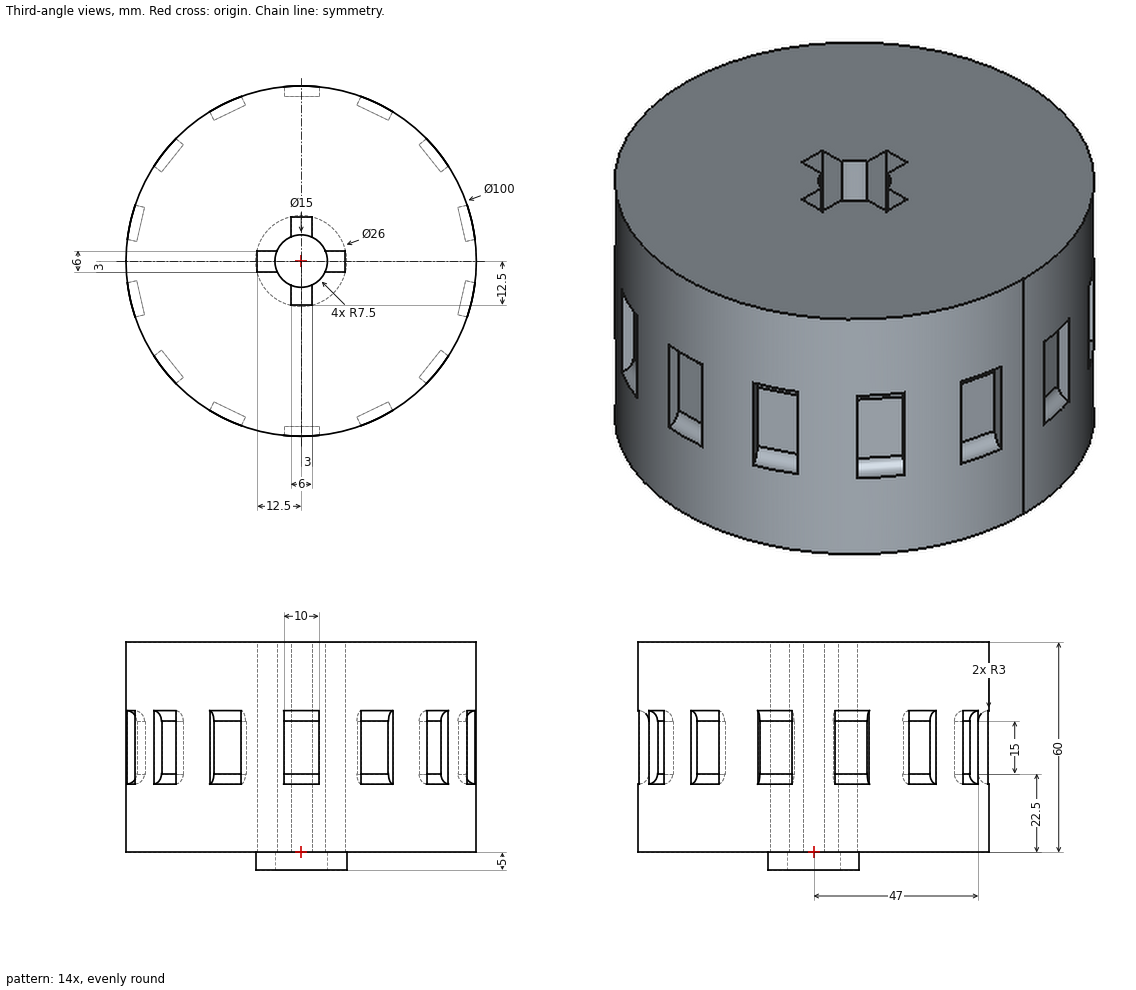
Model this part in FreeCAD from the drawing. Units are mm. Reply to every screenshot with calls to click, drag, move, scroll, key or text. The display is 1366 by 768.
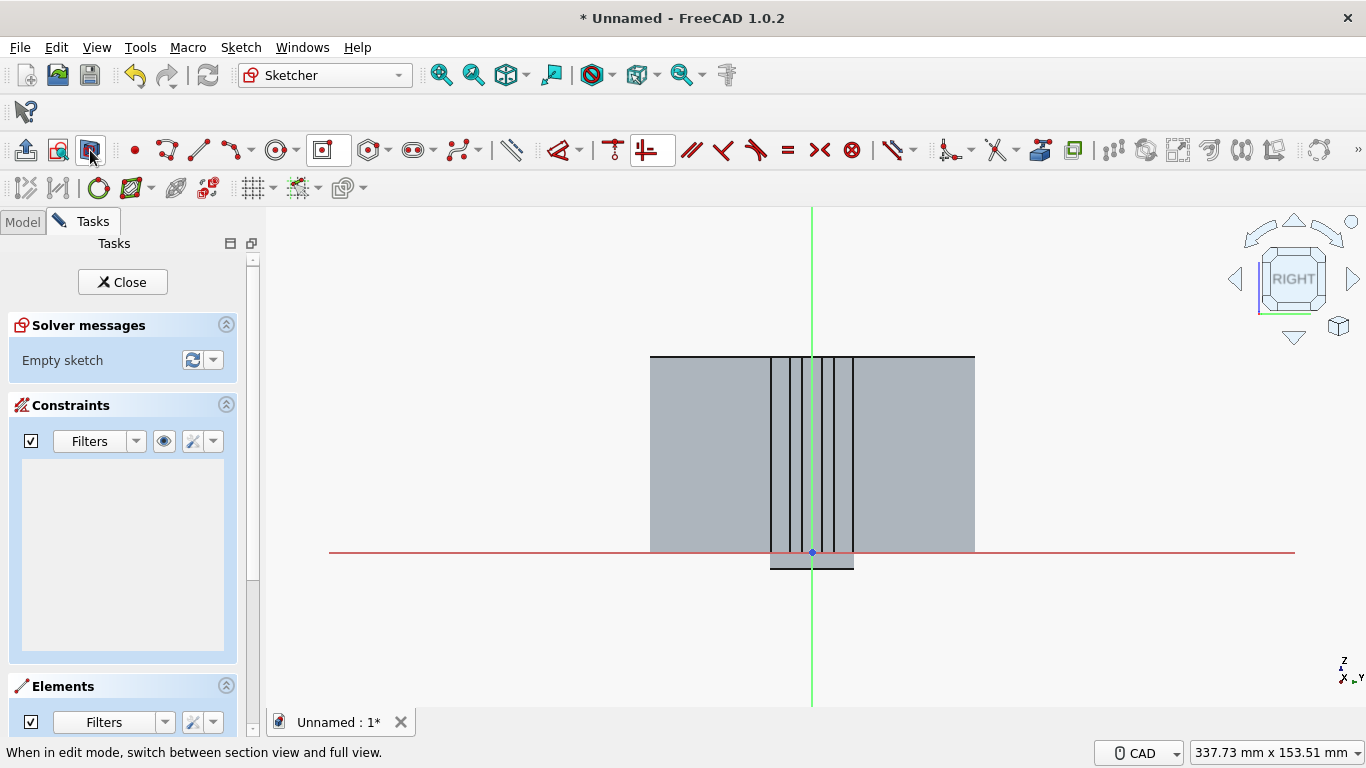
scroll(1032, 455, up, 8)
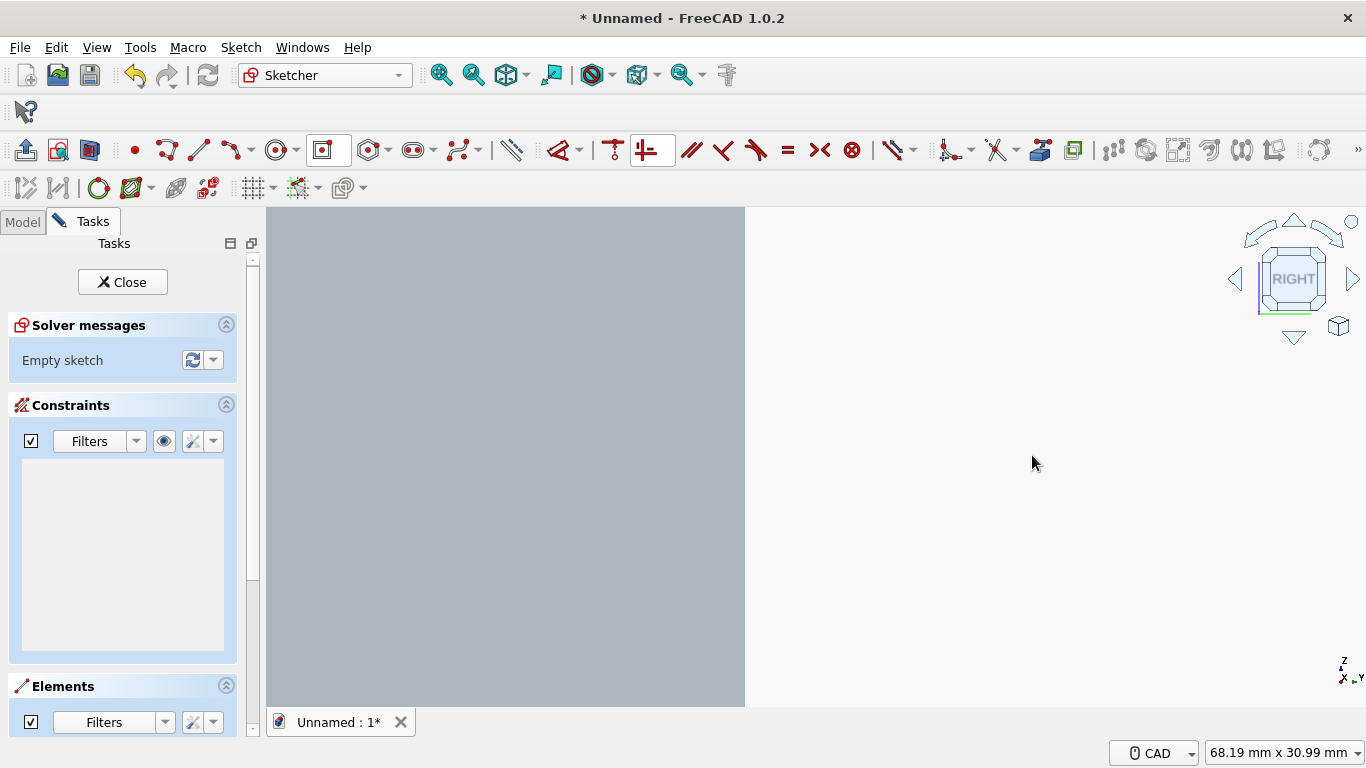
click(414, 150)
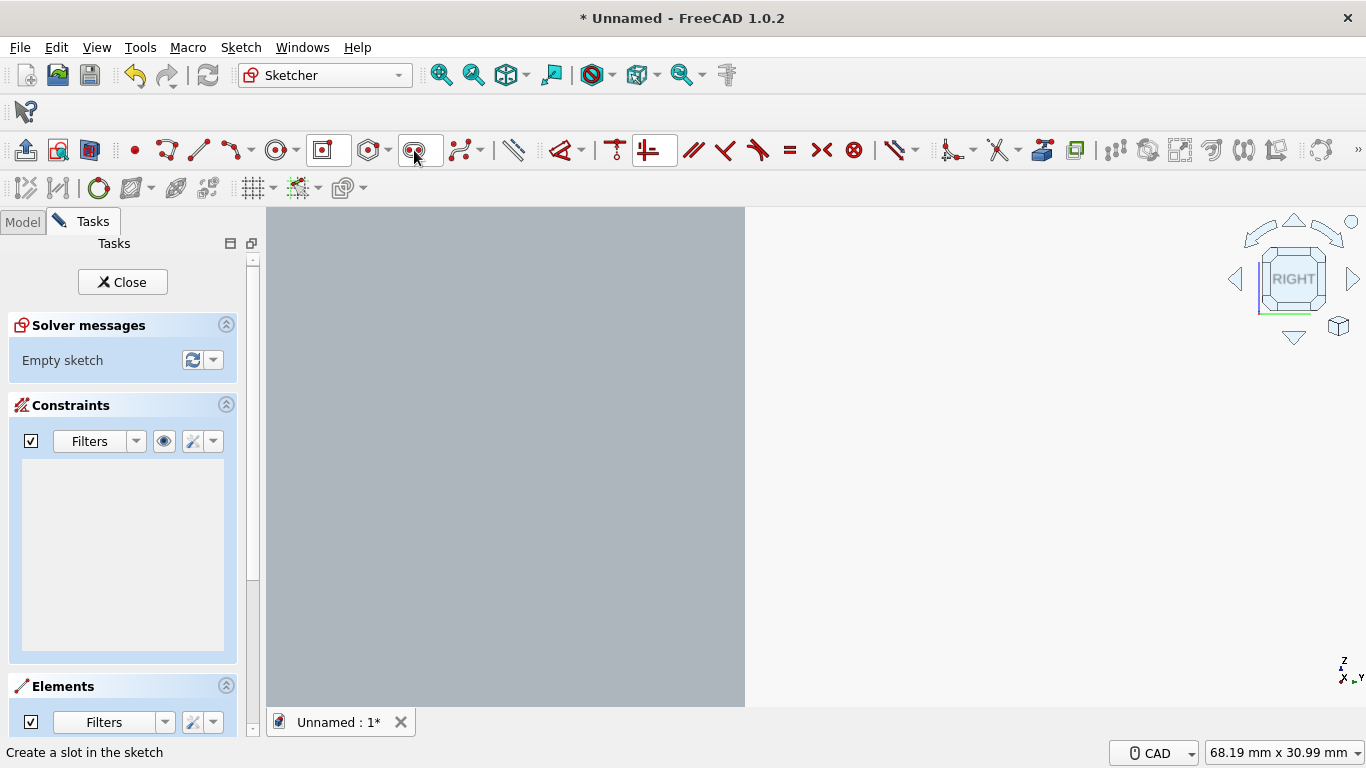
click(747, 575)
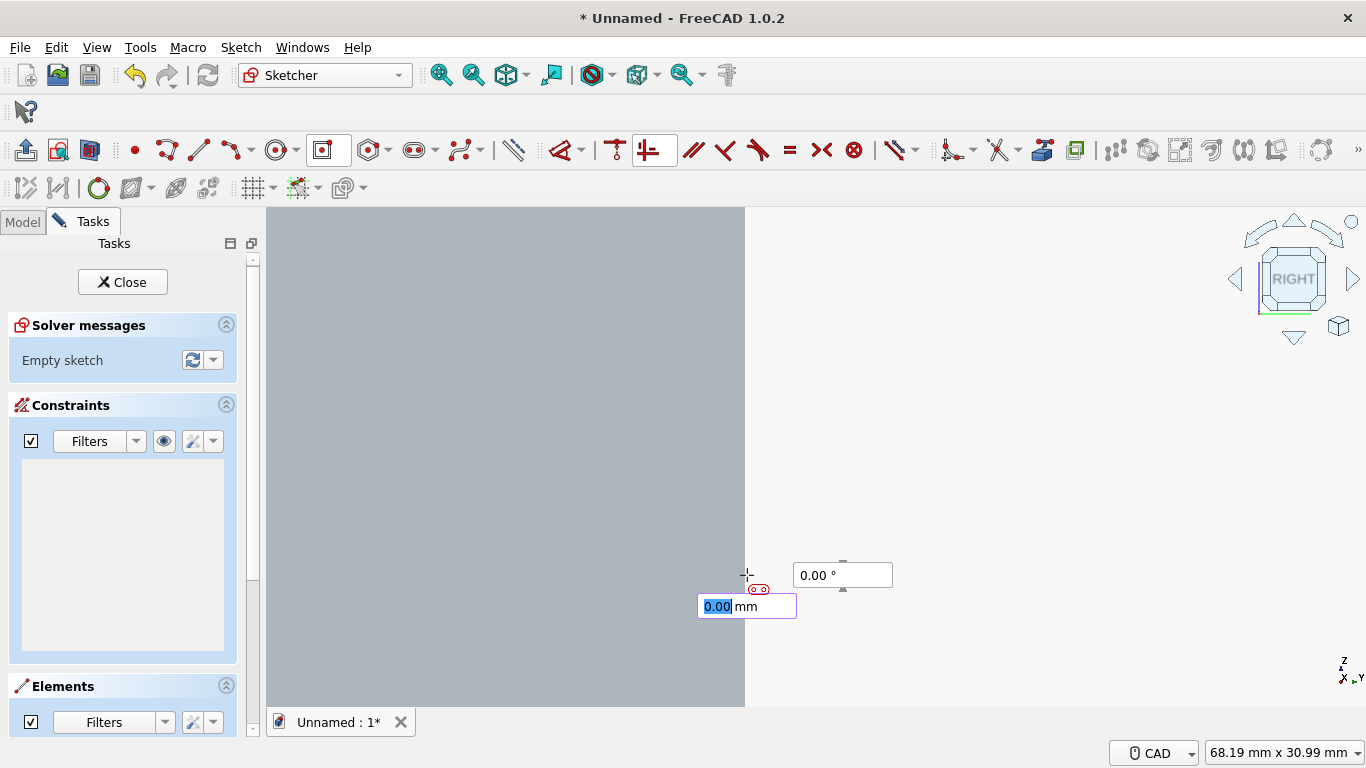
click(747, 333)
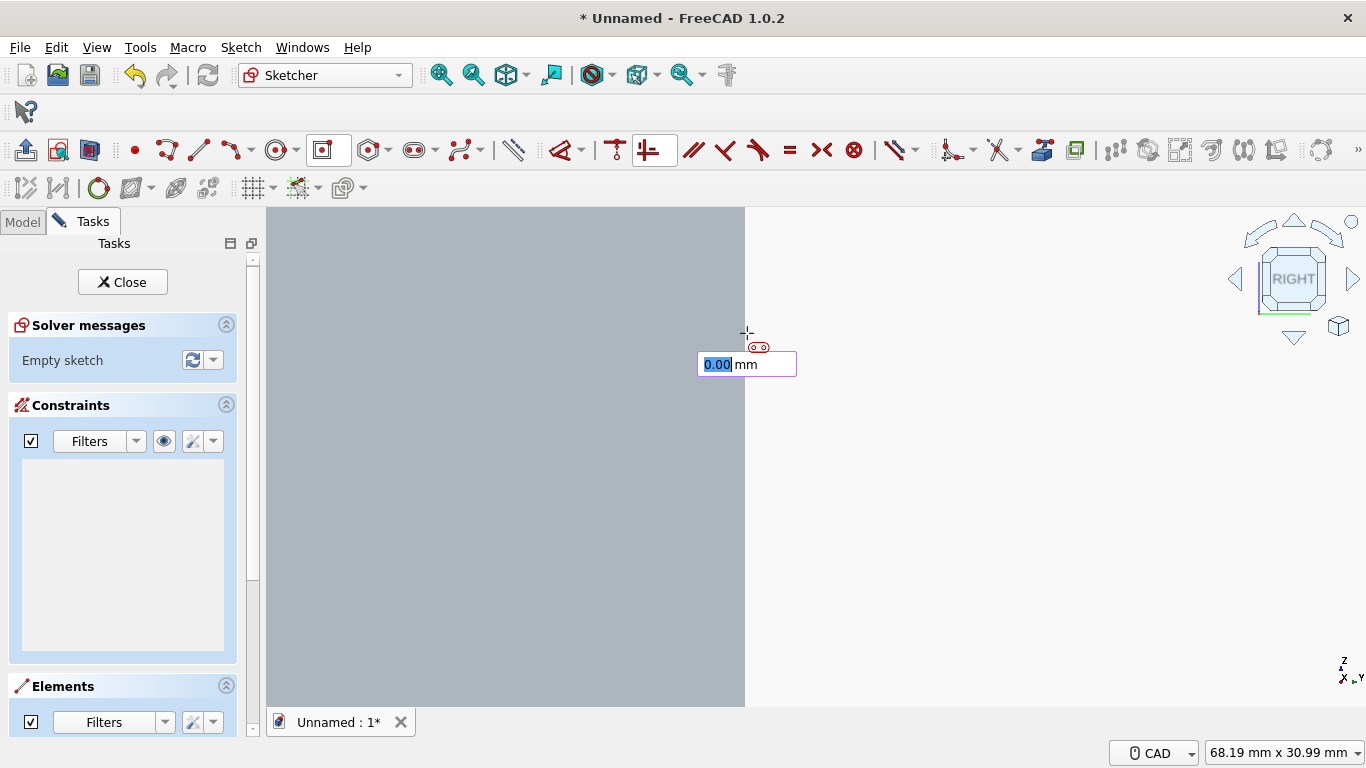
click(795, 454)
key(Escape)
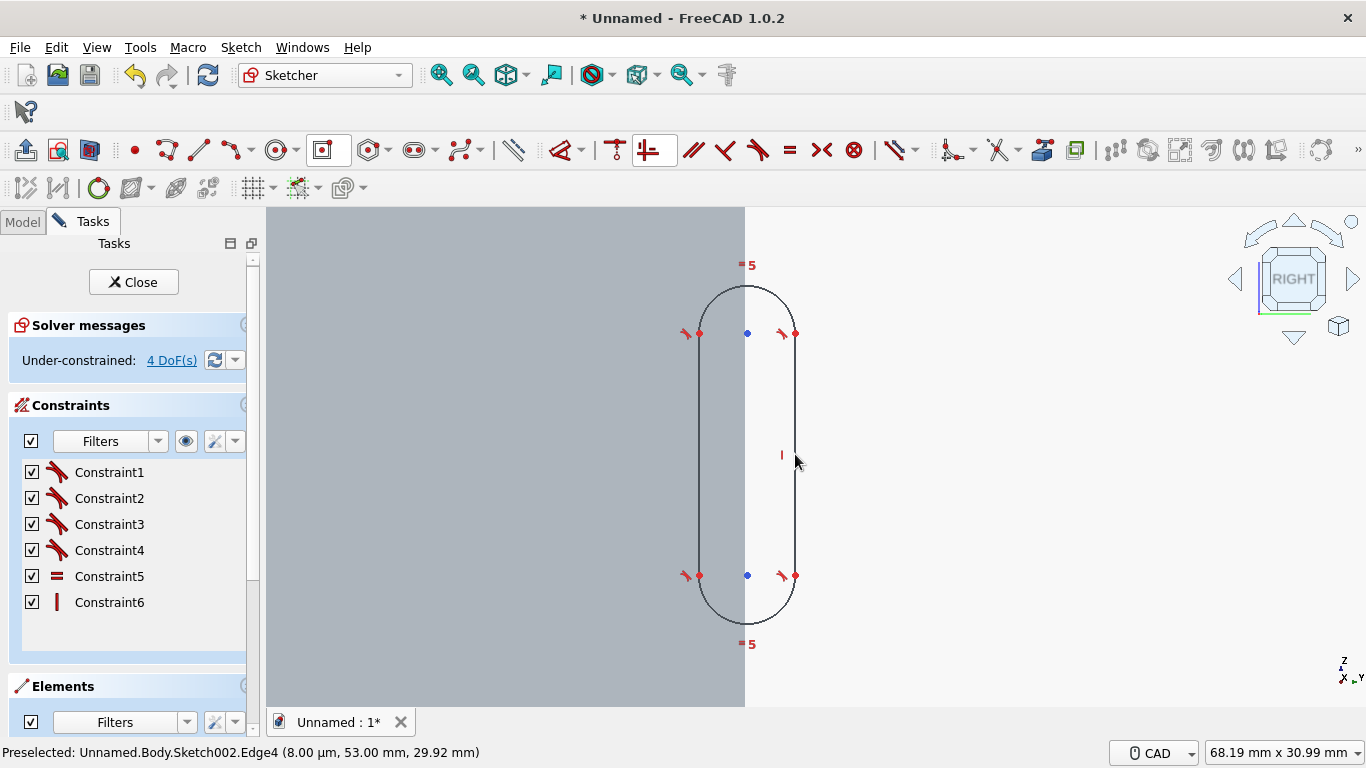
key(d)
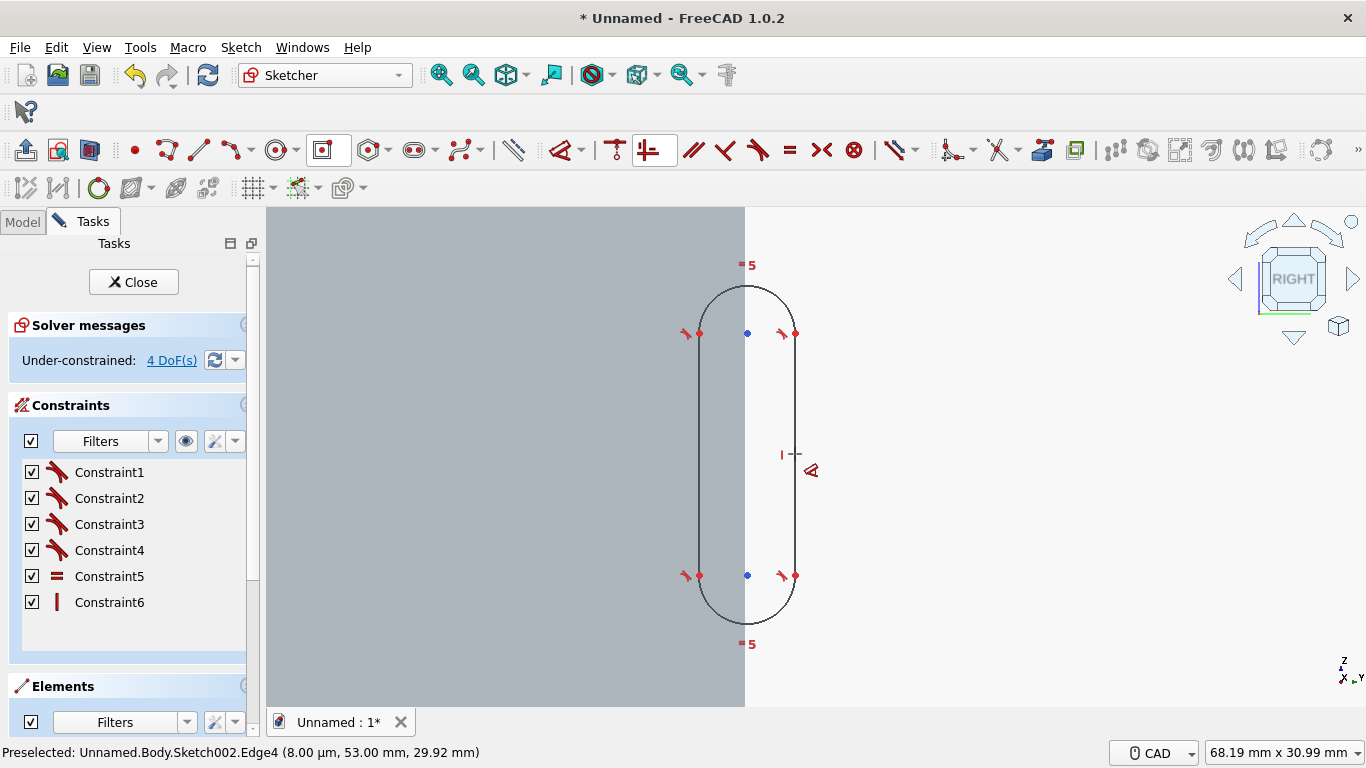
click(719, 615)
click(700, 641)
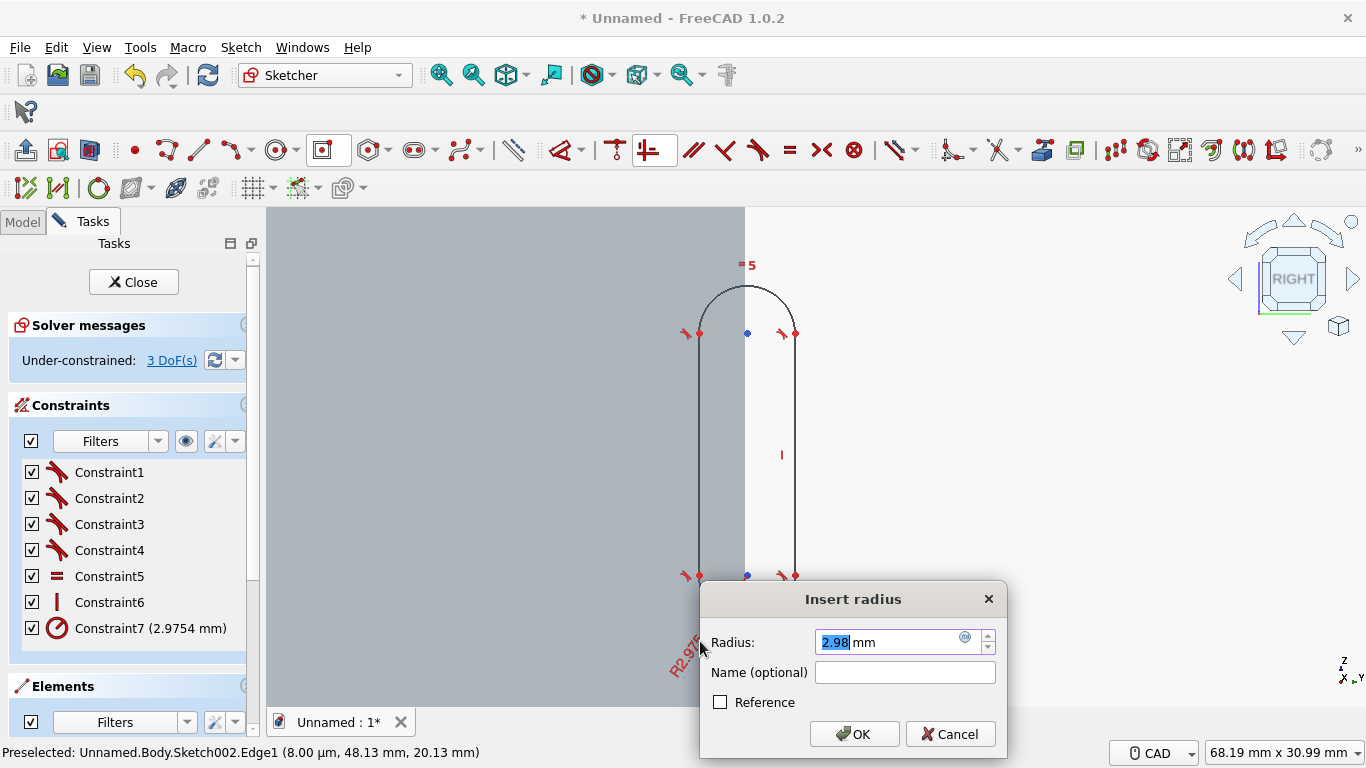
text(3)
key(Return)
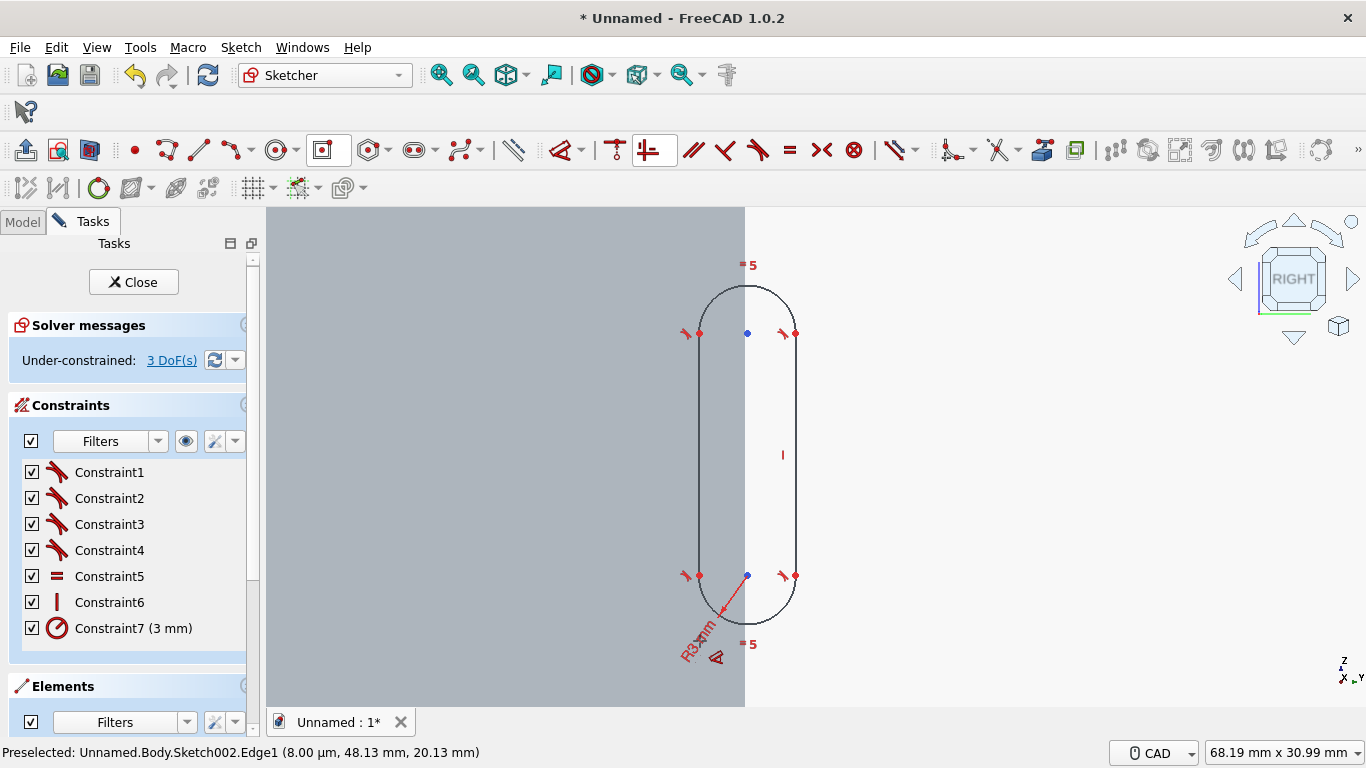
click(699, 503)
click(665, 455)